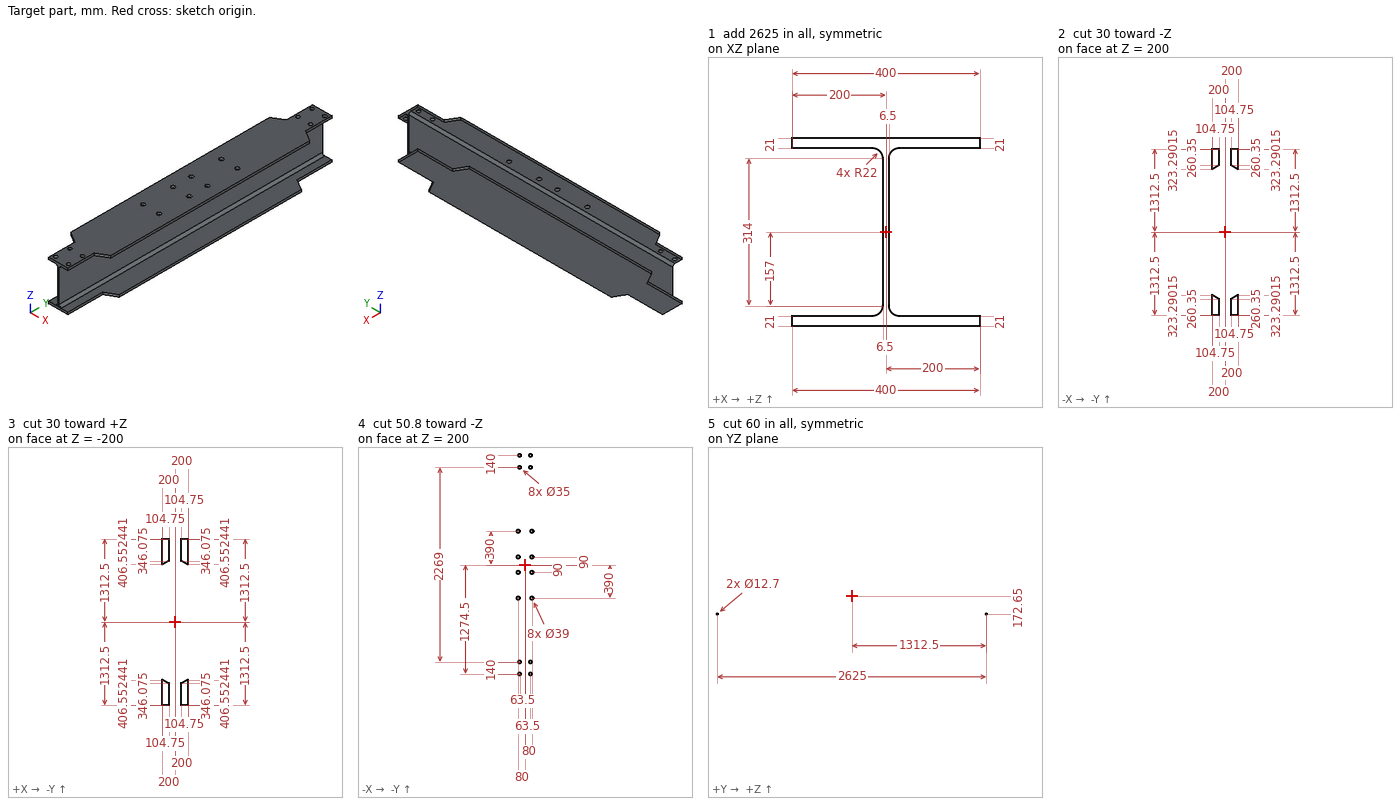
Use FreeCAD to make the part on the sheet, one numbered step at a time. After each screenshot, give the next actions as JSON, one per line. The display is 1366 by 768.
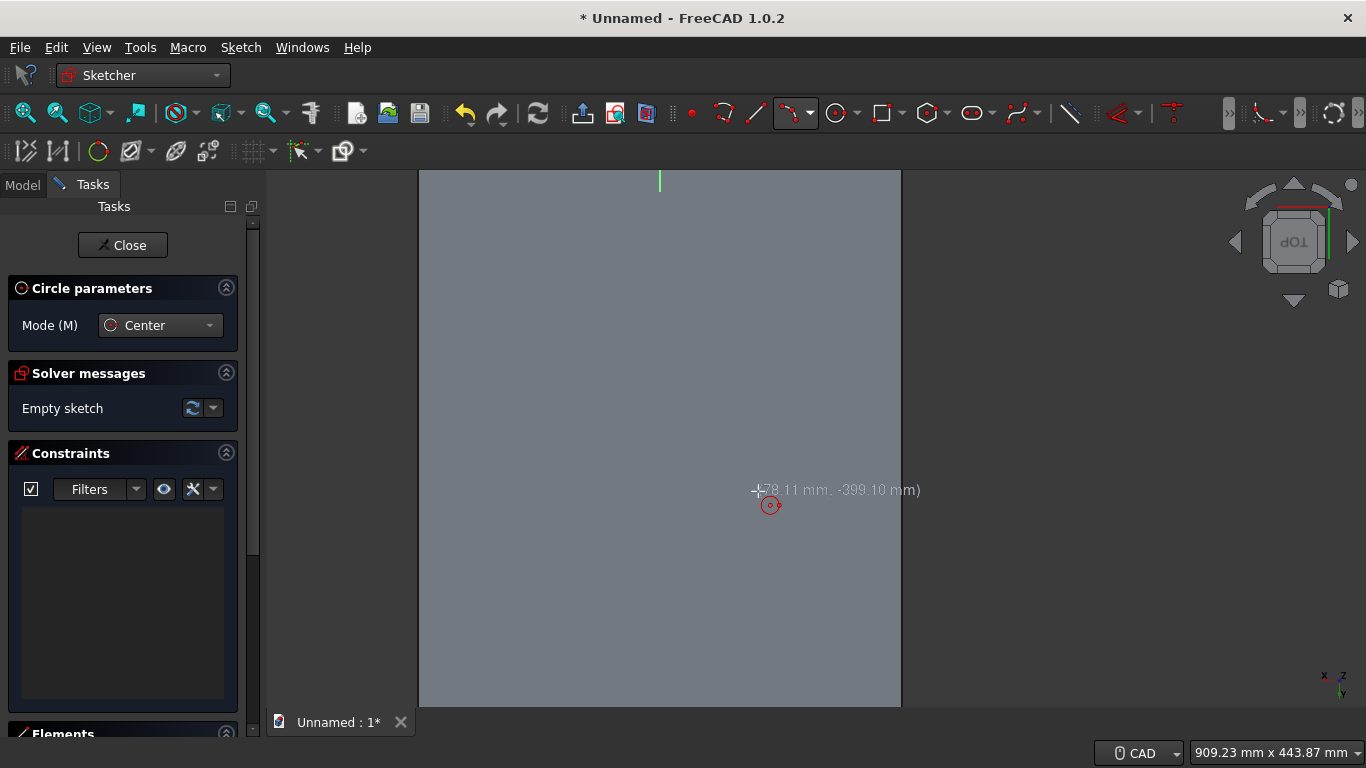
{"action": "scroll", "coordinate": [758, 492], "scroll_direction": "down", "scroll_amount": 11}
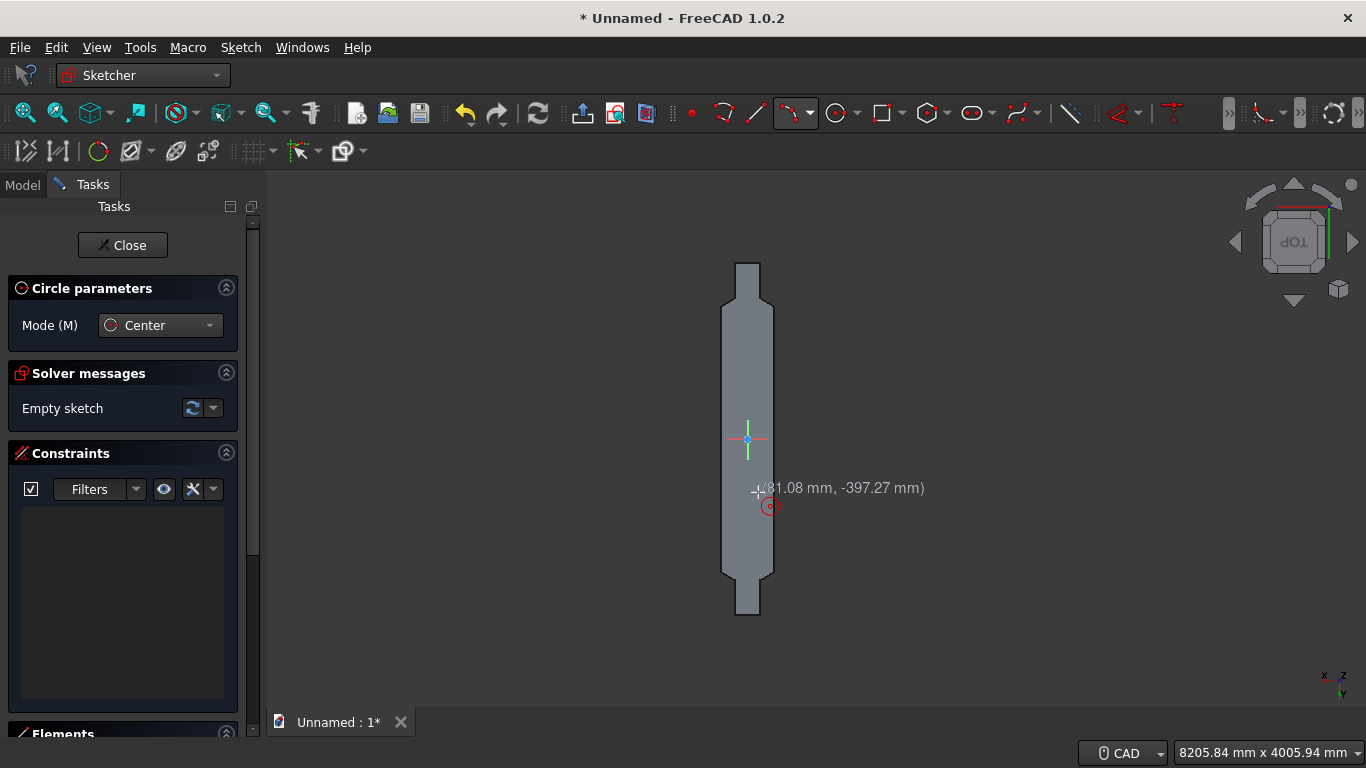
{"action": "scroll", "coordinate": [758, 492], "scroll_direction": "up", "scroll_amount": 2}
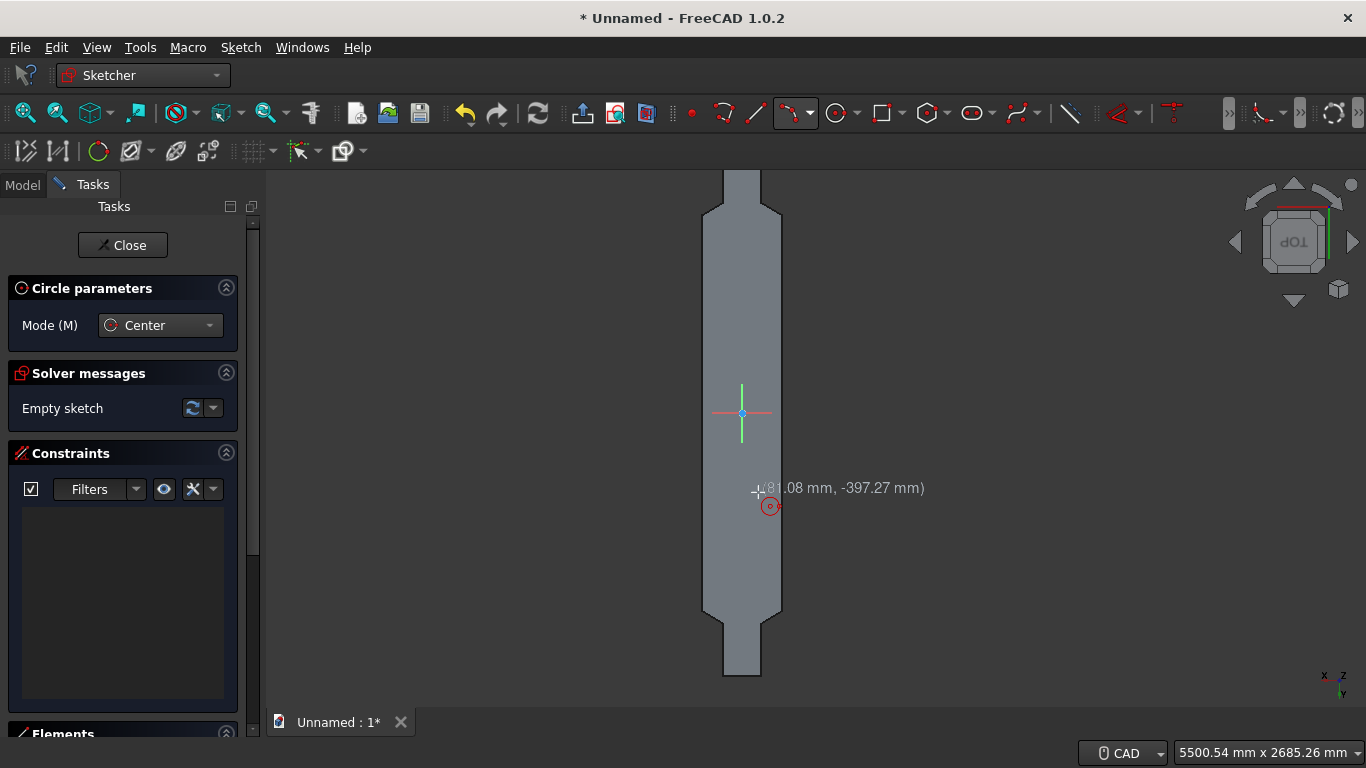
{"action": "left_click", "coordinate": [758, 491]}
{"action": "mouse_move", "coordinate": [761, 488]}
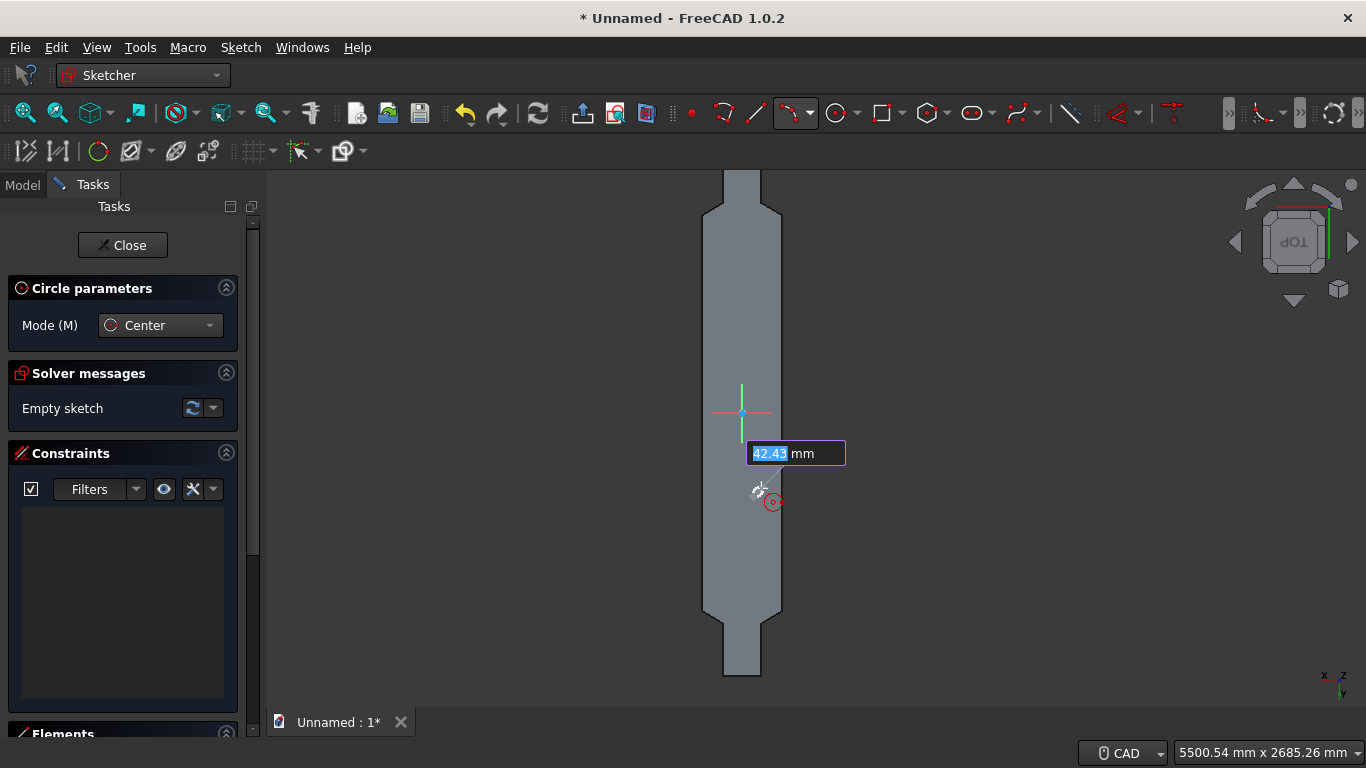
{"action": "type", "text": "39"}
{"action": "key", "text": "Return"}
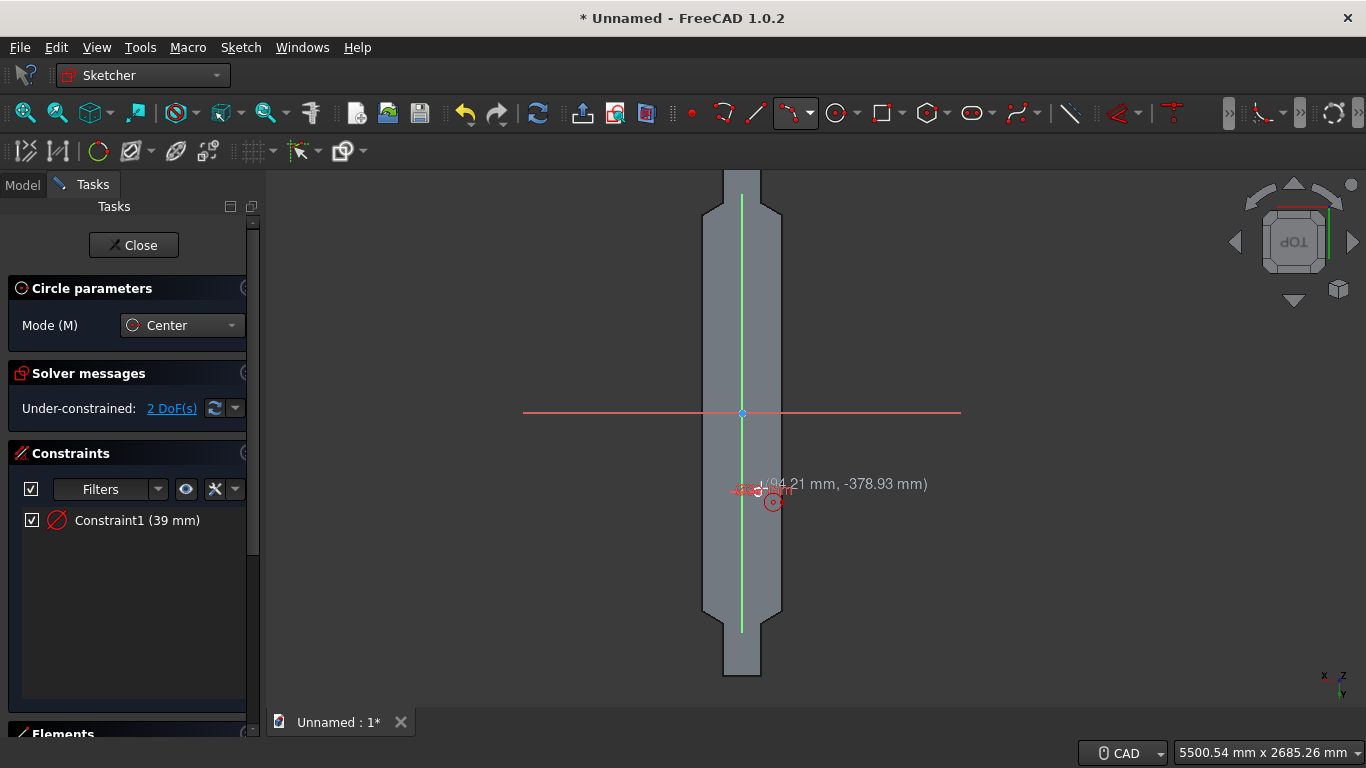
{"action": "scroll", "coordinate": [726, 491], "scroll_direction": "up", "scroll_amount": 9}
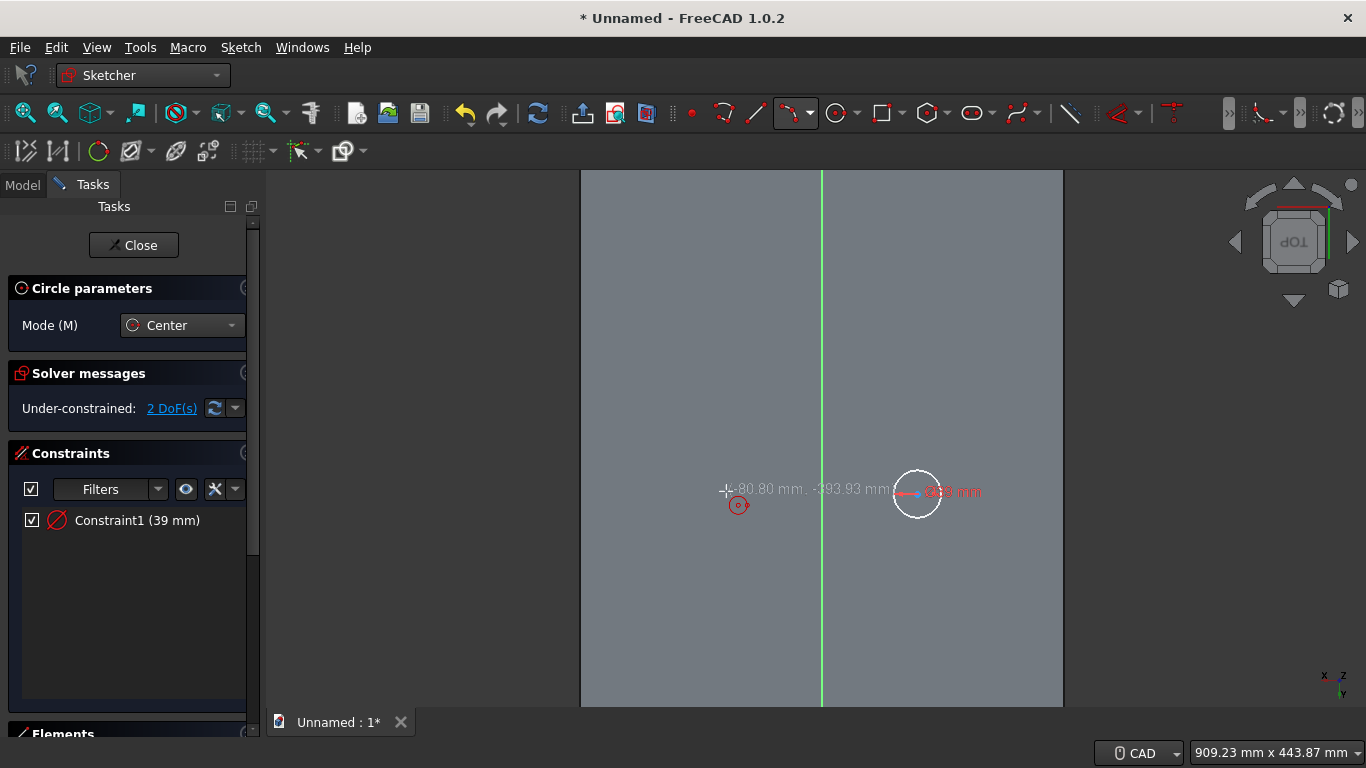
{"action": "scroll", "coordinate": [738, 491], "scroll_direction": "down", "scroll_amount": 11}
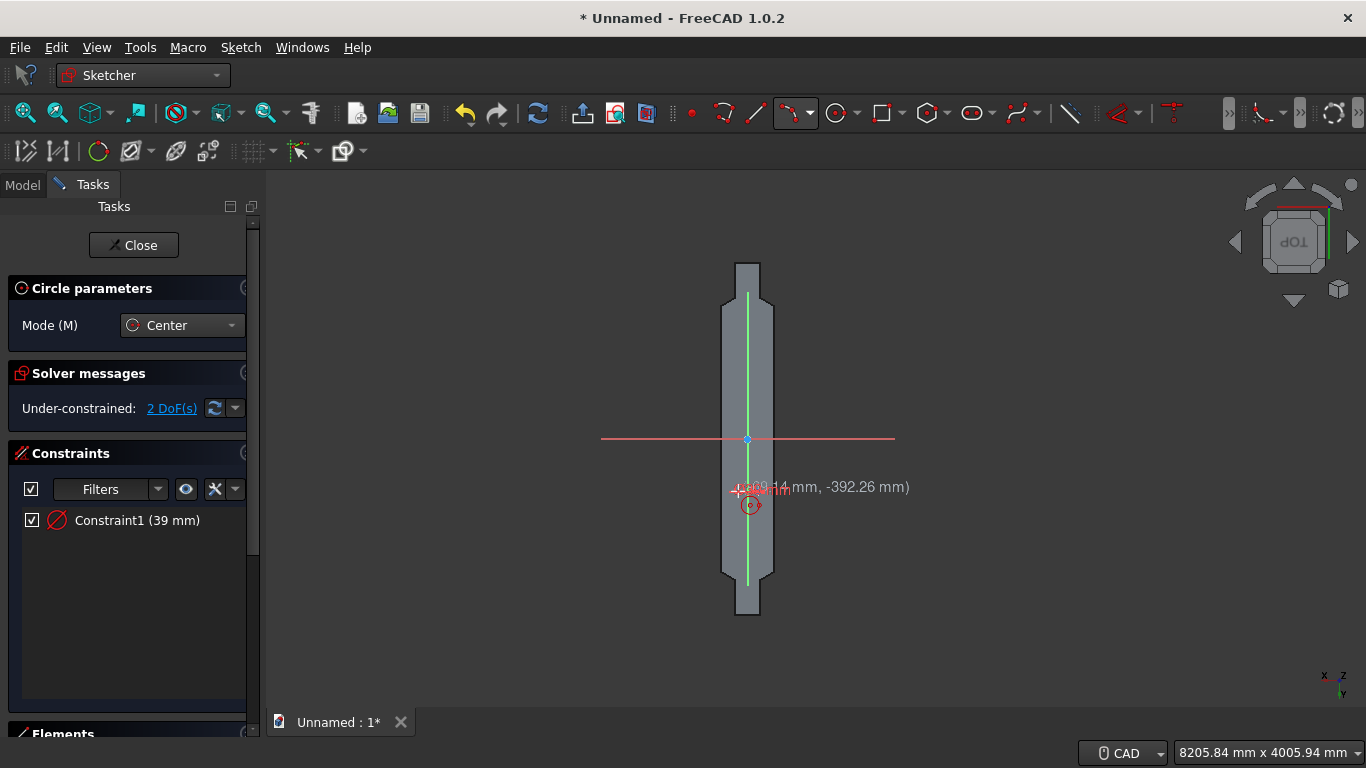
{"action": "scroll", "coordinate": [737, 491], "scroll_direction": "up", "scroll_amount": 2}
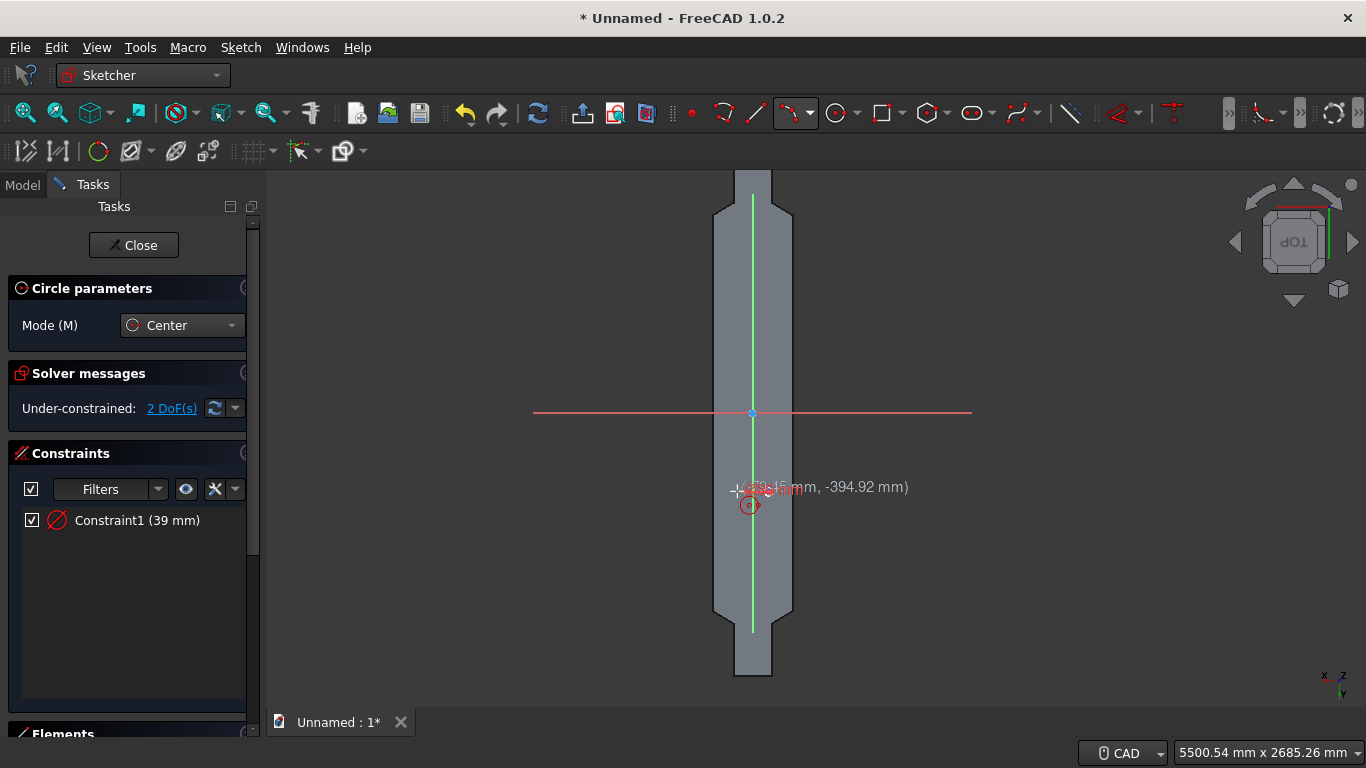
{"action": "left_click", "coordinate": [737, 491]}
{"action": "mouse_move", "coordinate": [734, 488]}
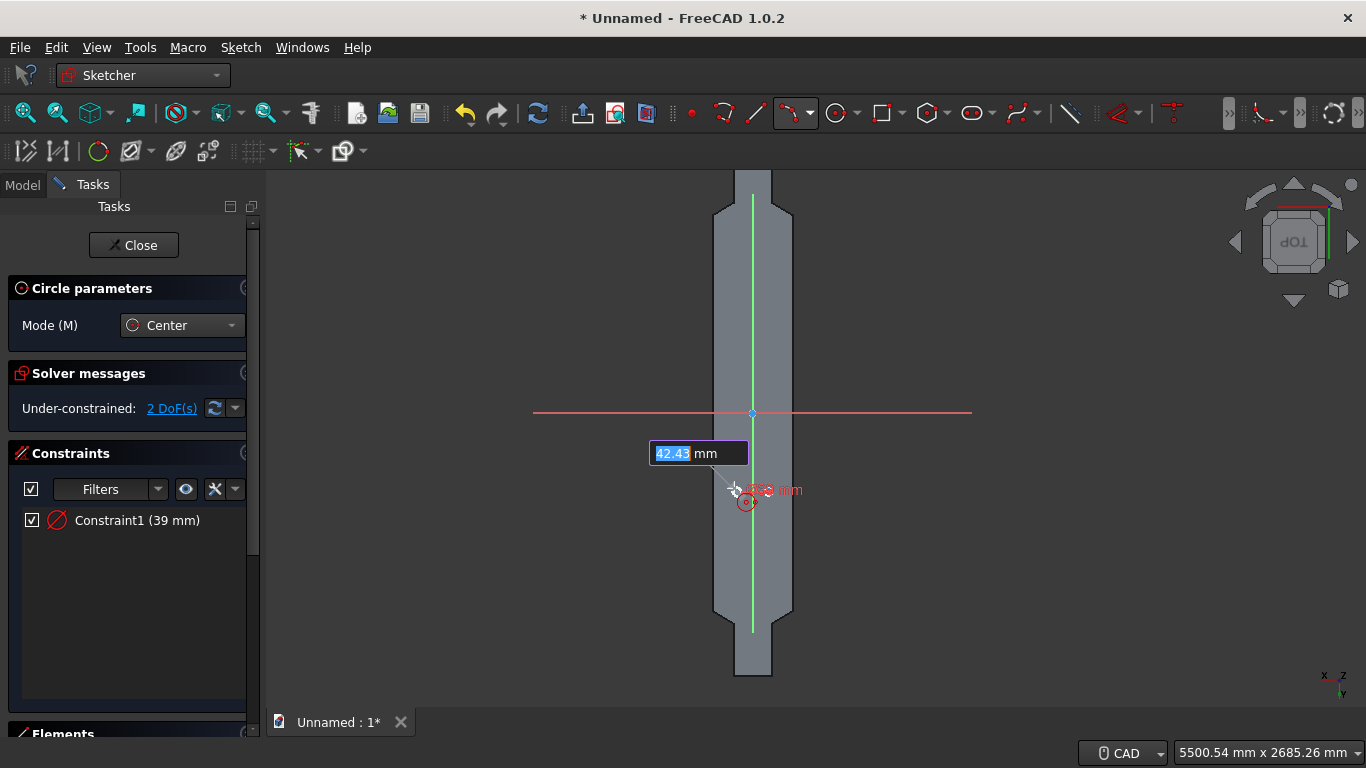
{"action": "type", "text": "39"}
{"action": "key", "text": "Return"}